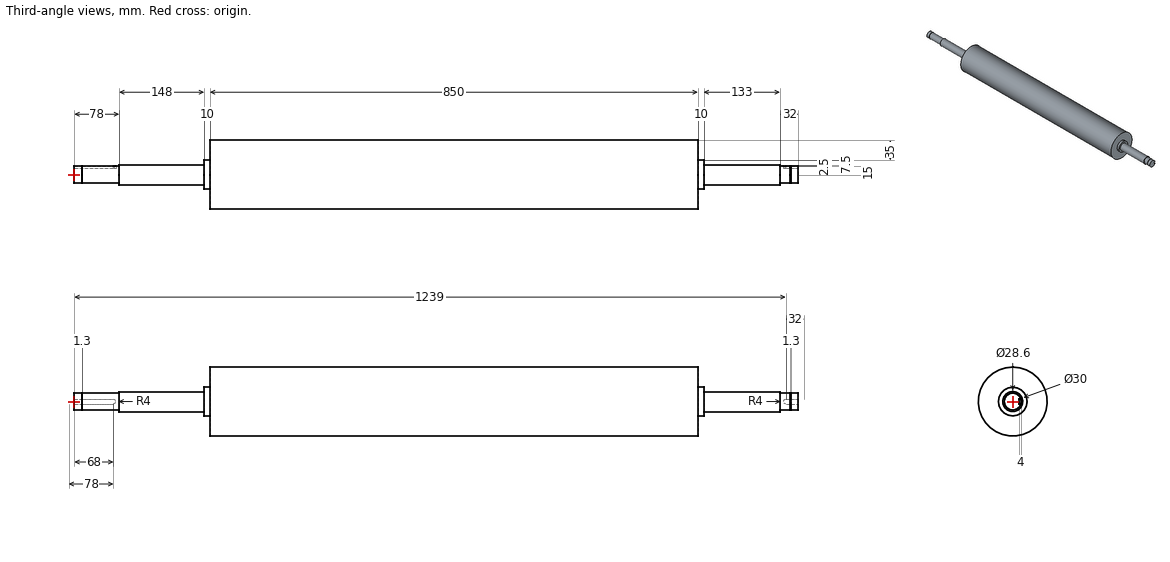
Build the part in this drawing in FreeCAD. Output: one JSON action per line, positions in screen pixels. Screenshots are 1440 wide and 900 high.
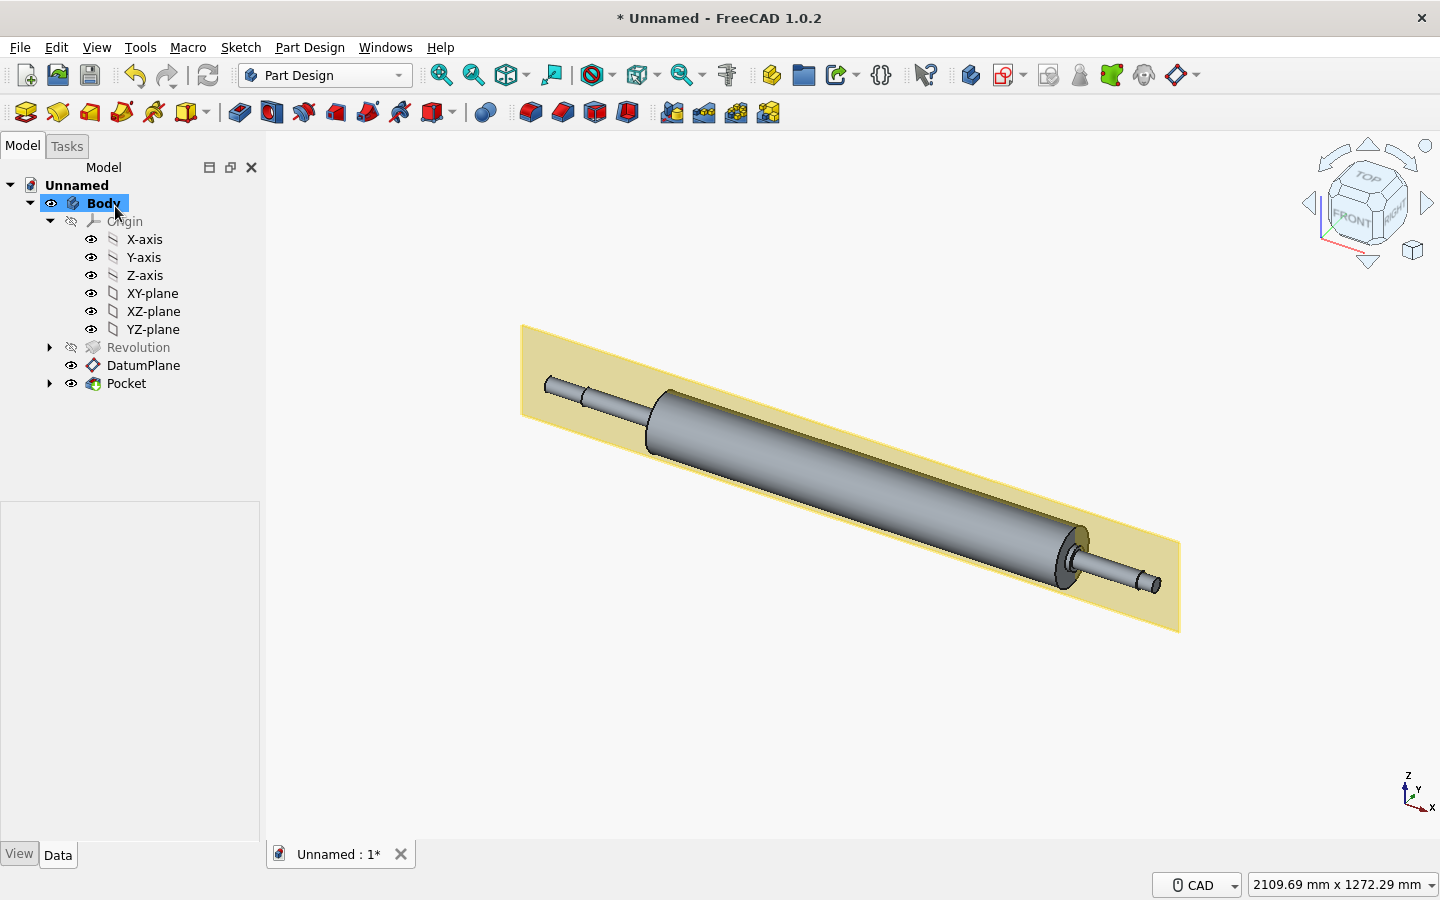
{"action": "left_click", "coordinate": [116, 365]}
{"action": "key", "text": "space"}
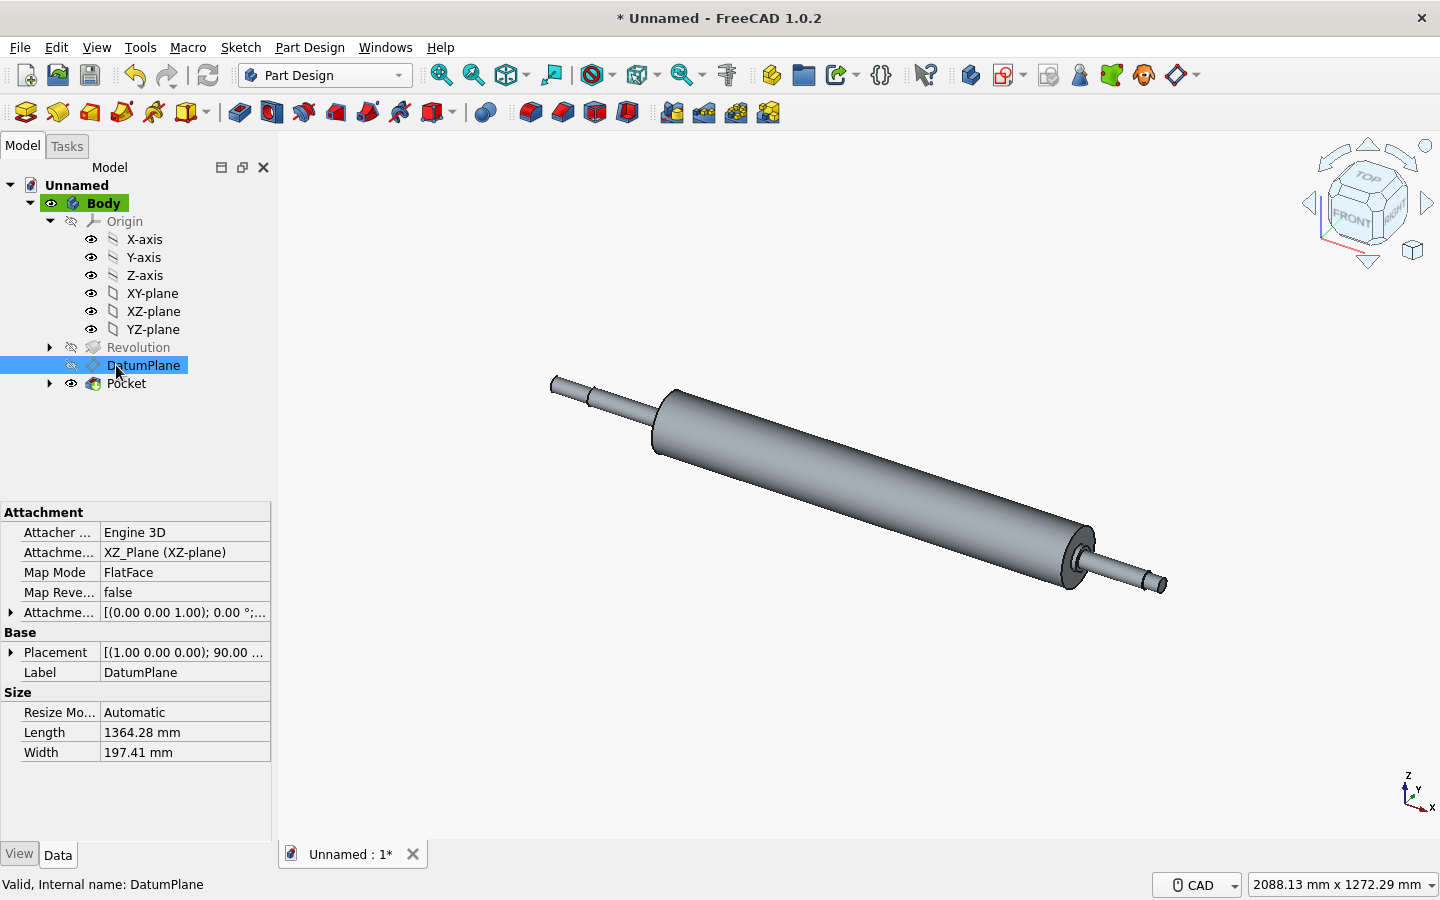
{"action": "left_click", "coordinate": [136, 329]}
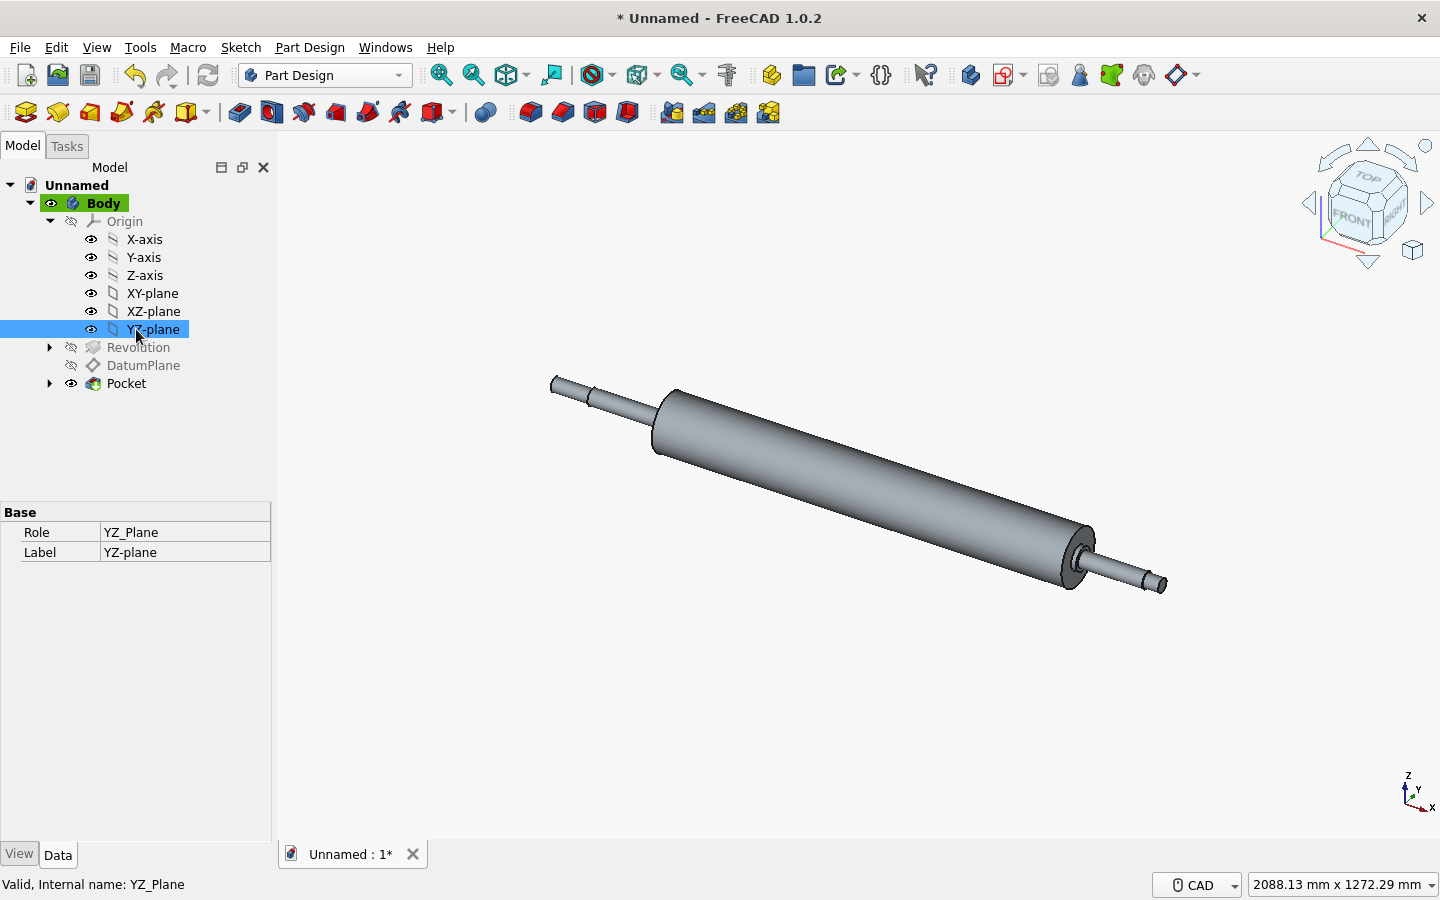
{"action": "left_click", "coordinate": [1176, 76]}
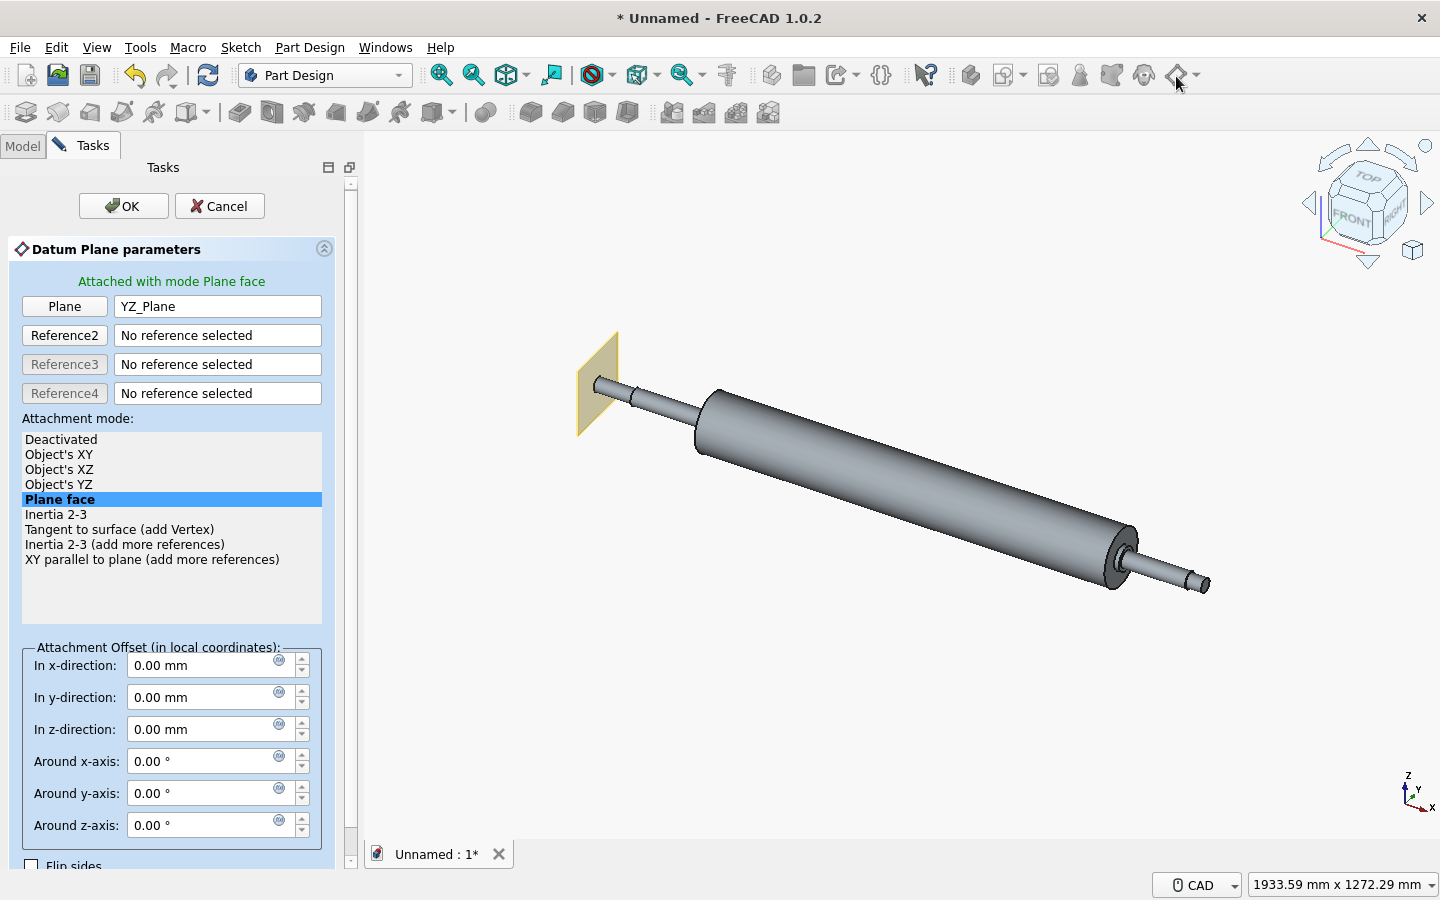
{"action": "triple_click", "coordinate": [210, 729]}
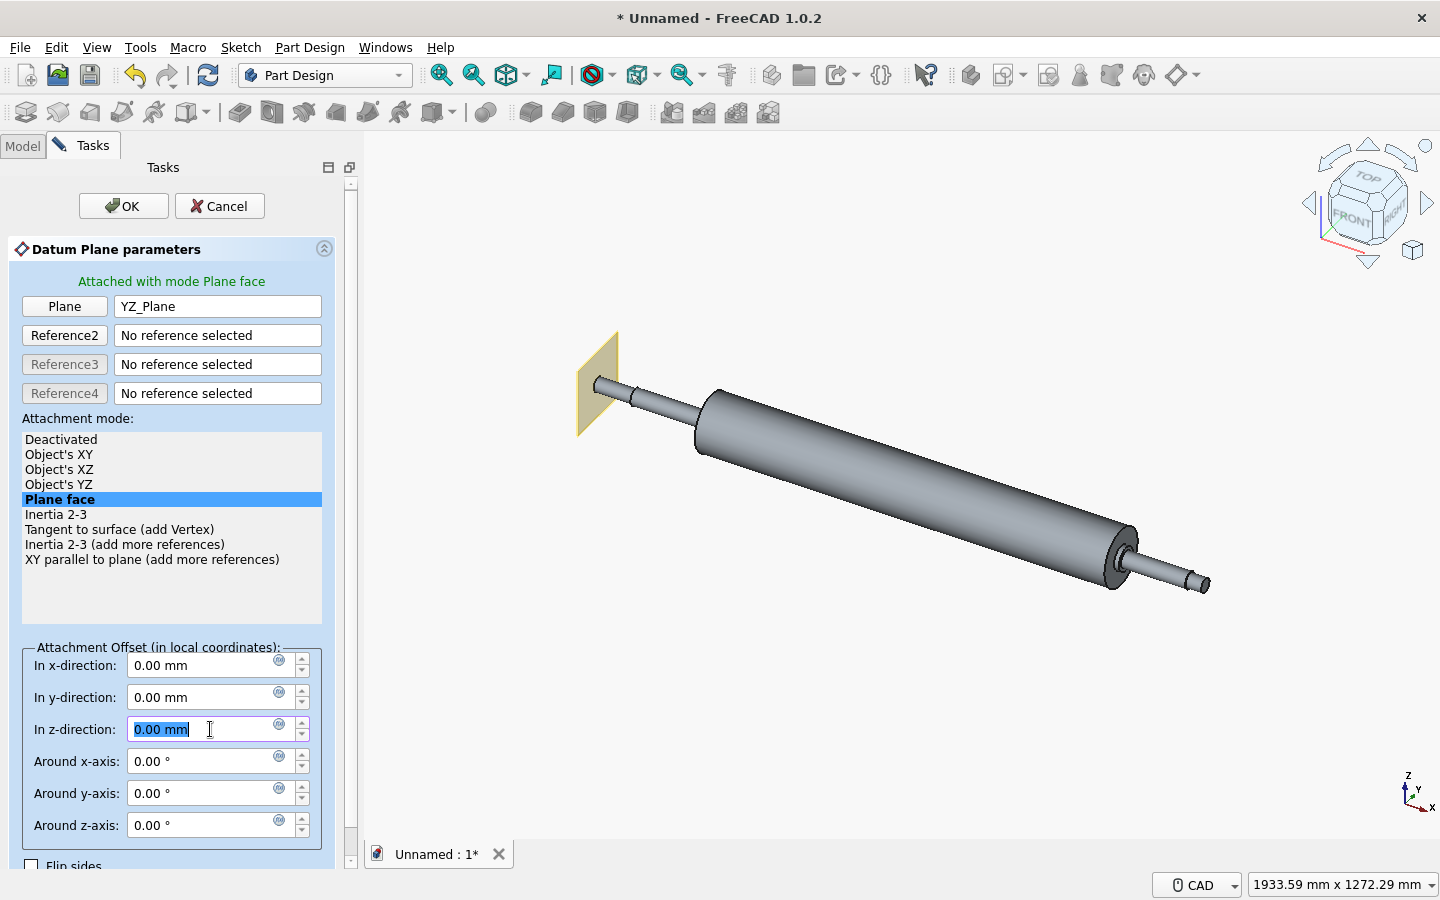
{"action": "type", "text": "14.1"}
{"action": "key", "text": "Tab"}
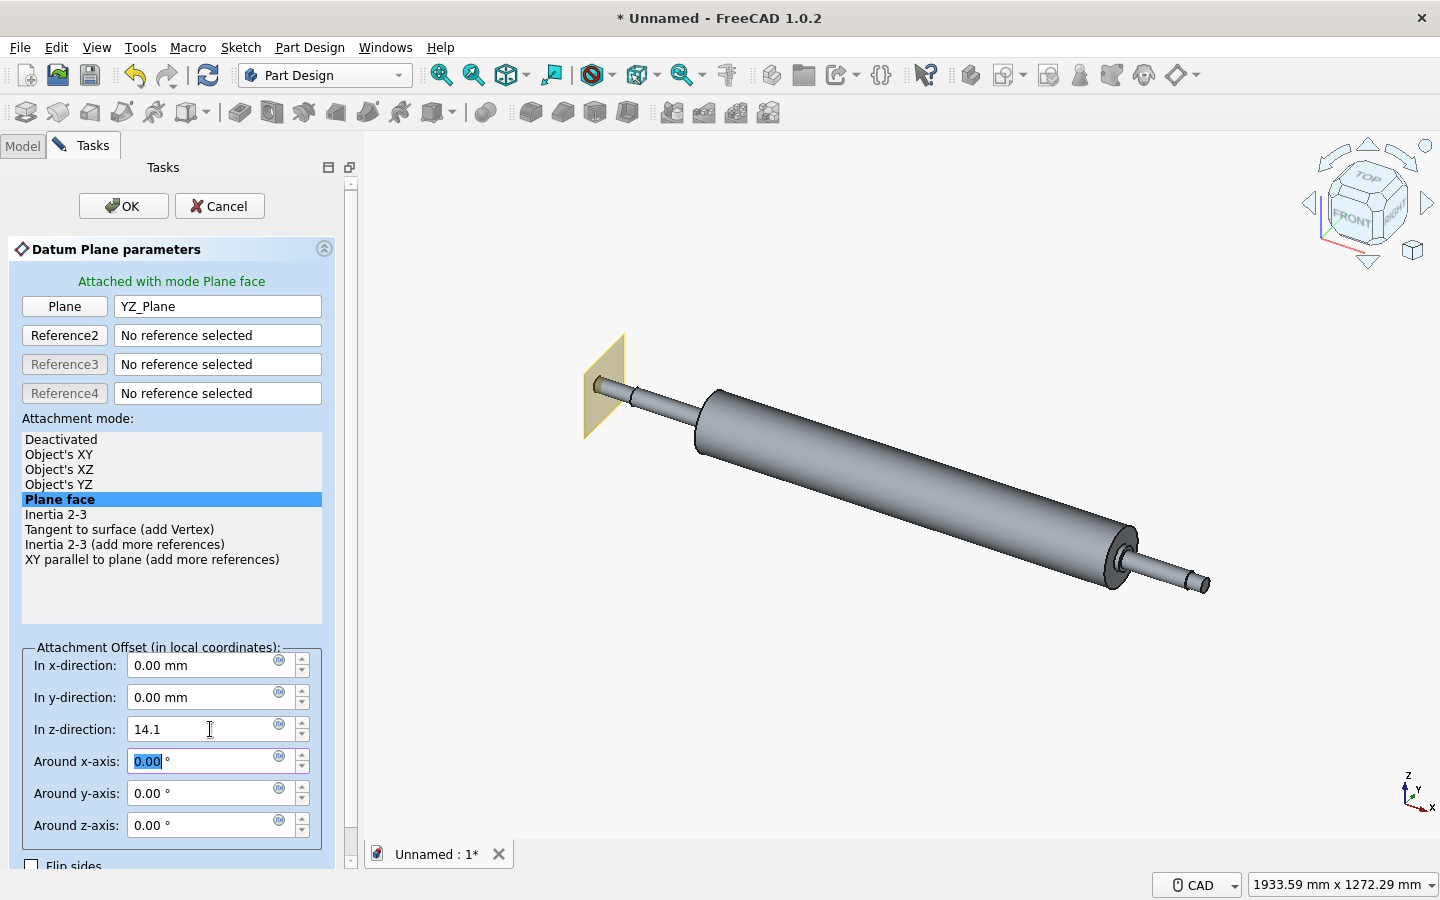
{"action": "left_click", "coordinate": [124, 206]}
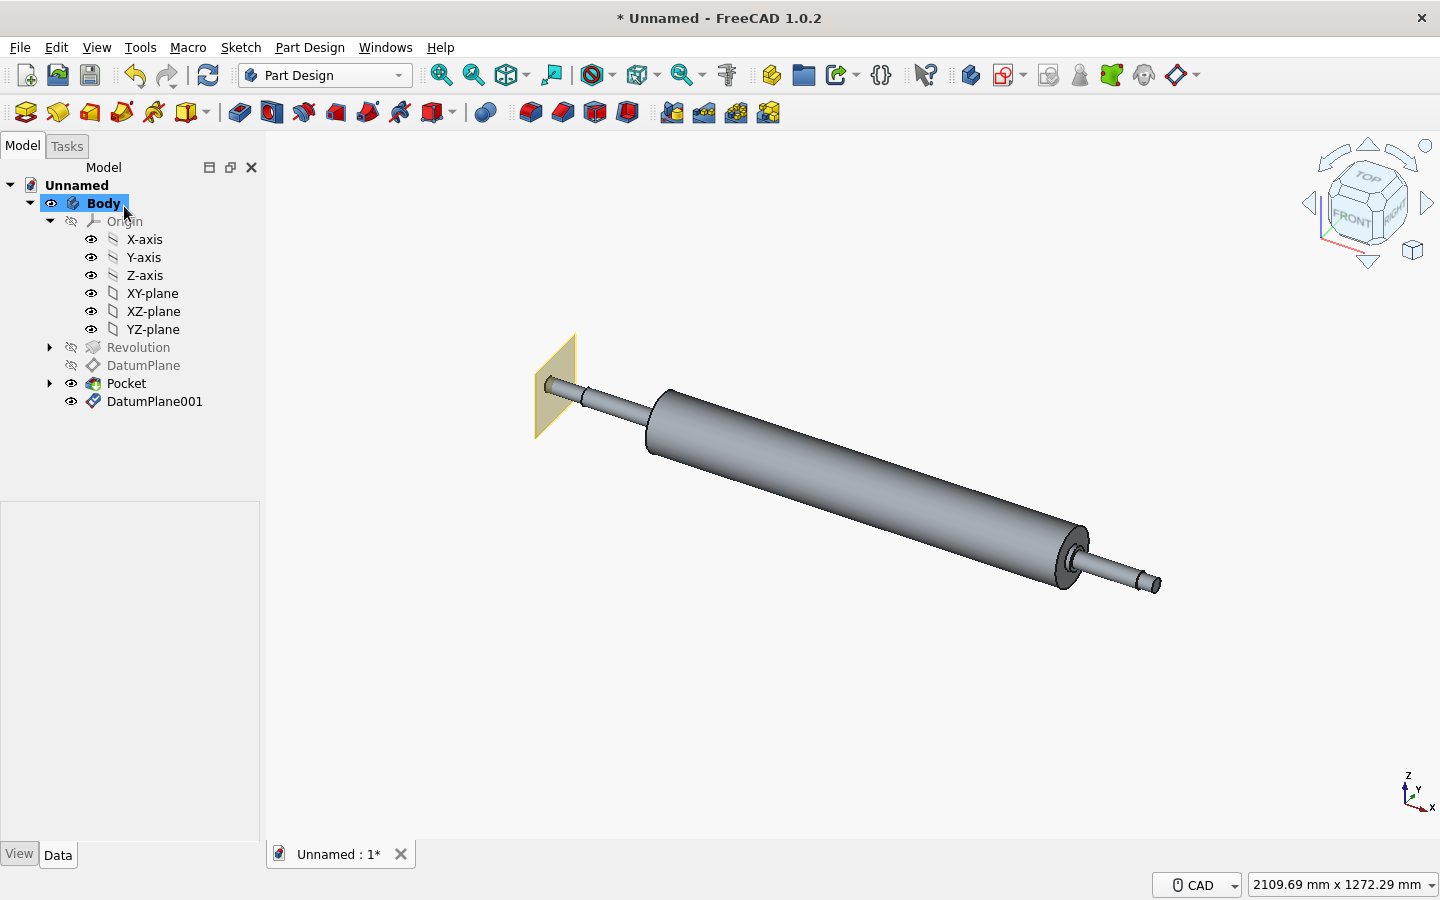
{"action": "left_click", "coordinate": [116, 401]}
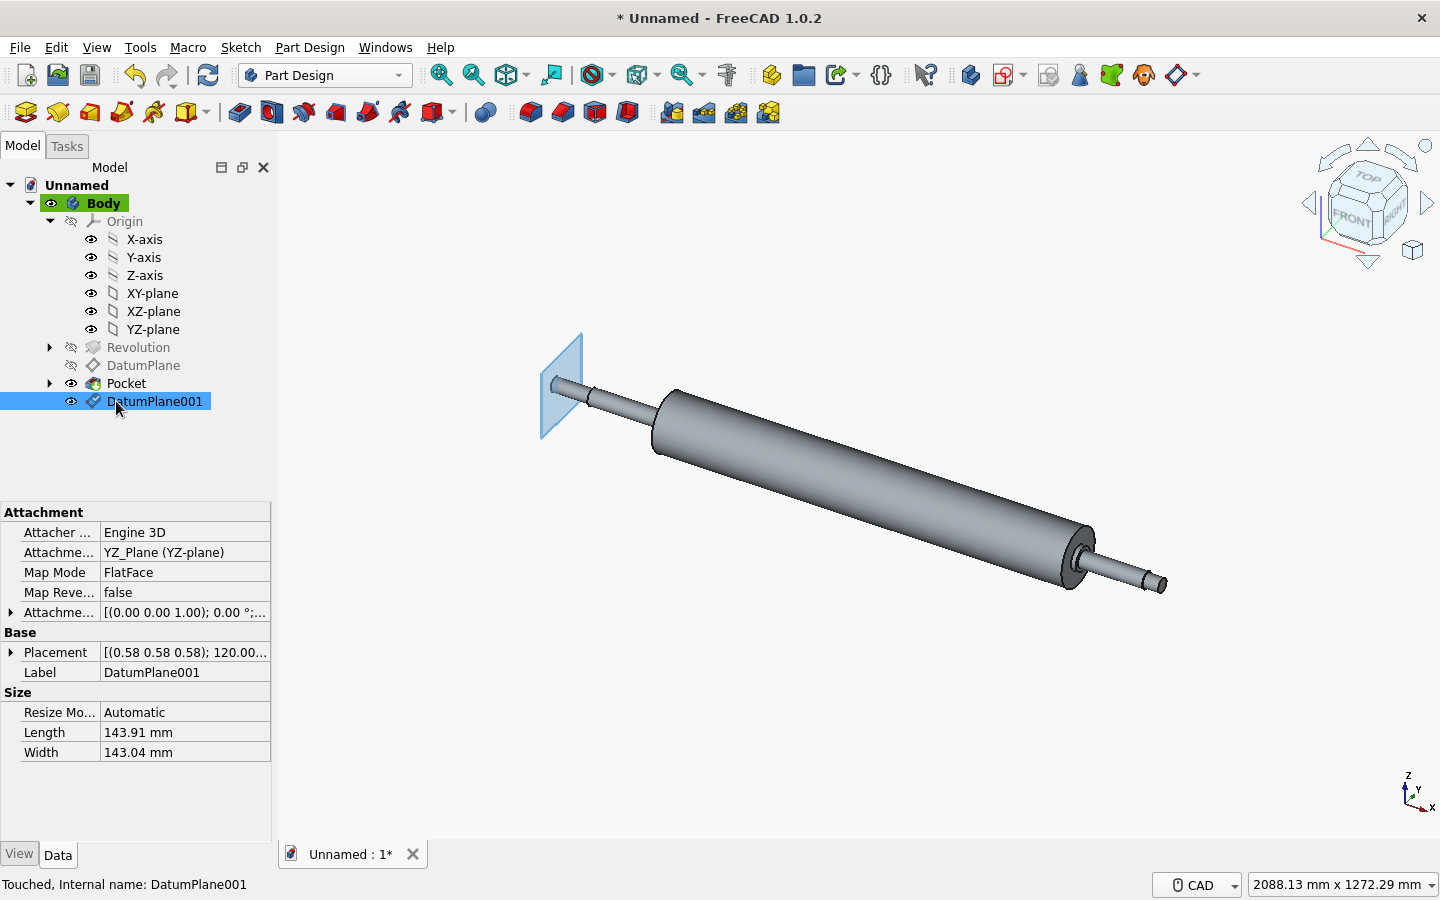
{"action": "left_click", "coordinate": [1004, 76]}